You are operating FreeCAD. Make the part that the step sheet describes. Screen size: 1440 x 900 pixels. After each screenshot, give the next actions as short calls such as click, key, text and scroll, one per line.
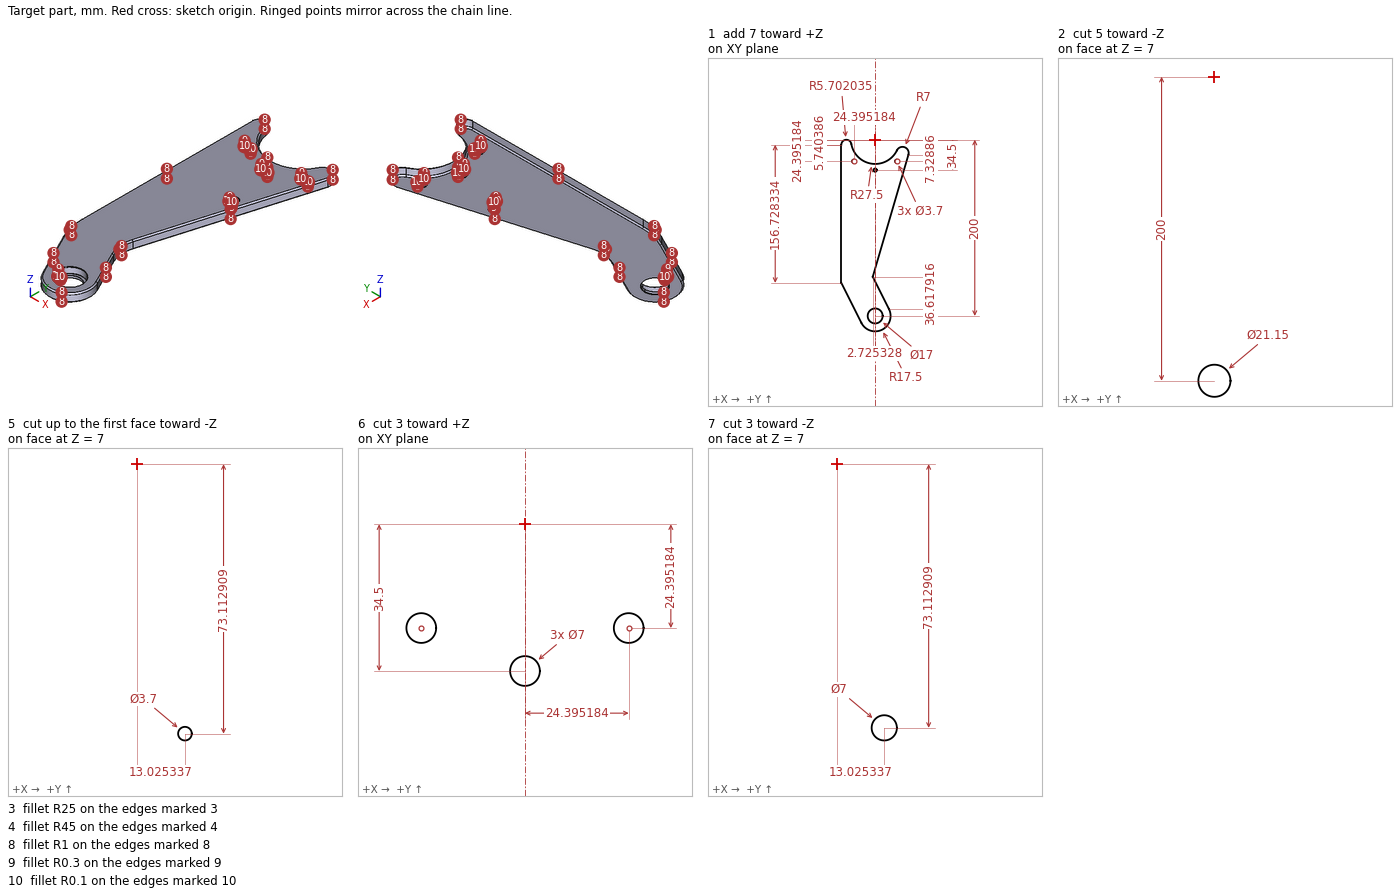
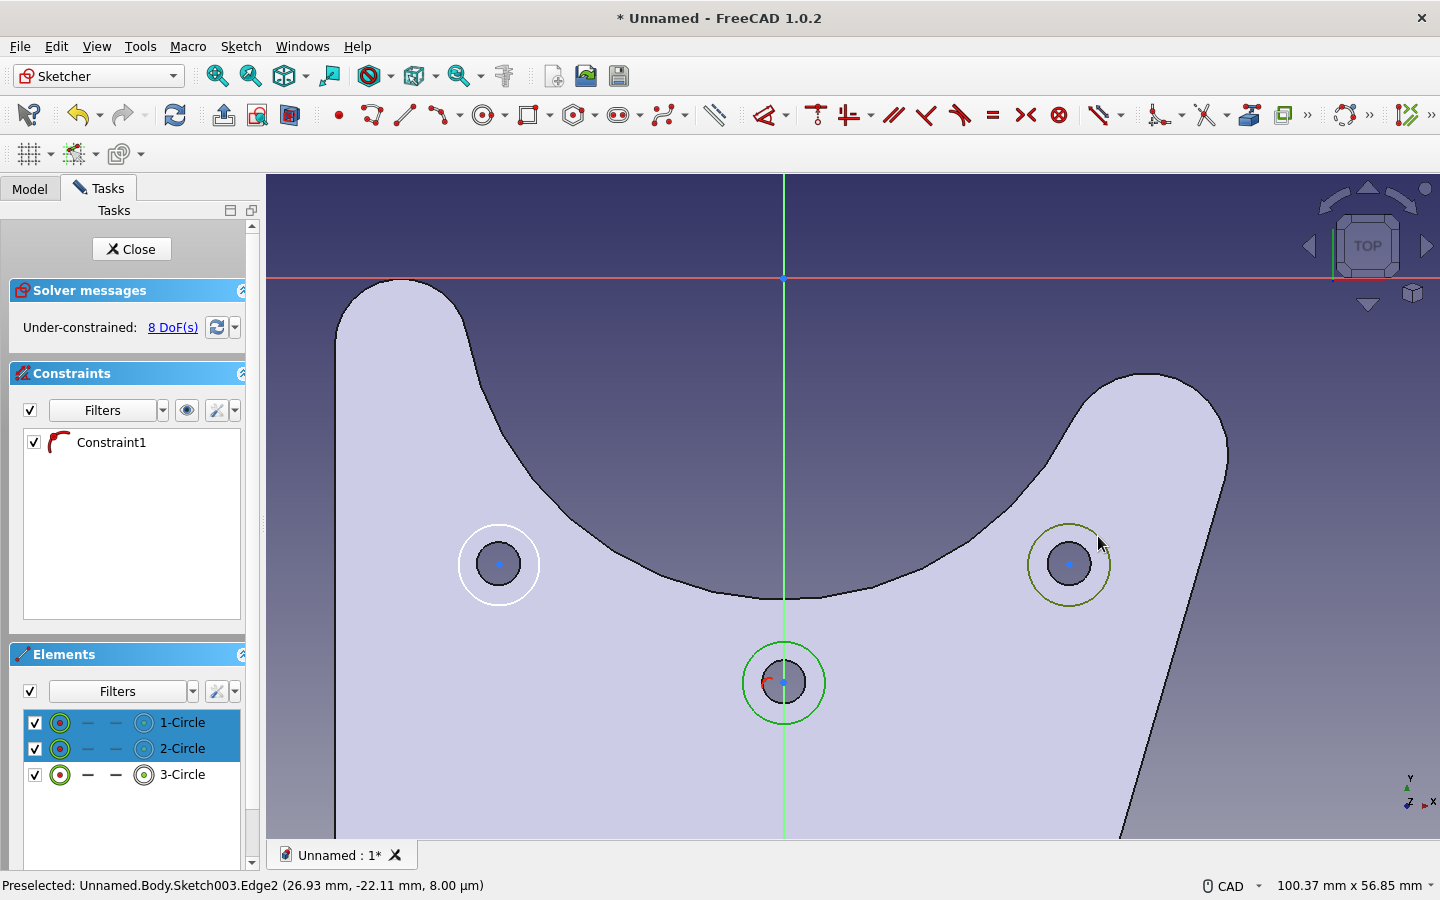
click(527, 536)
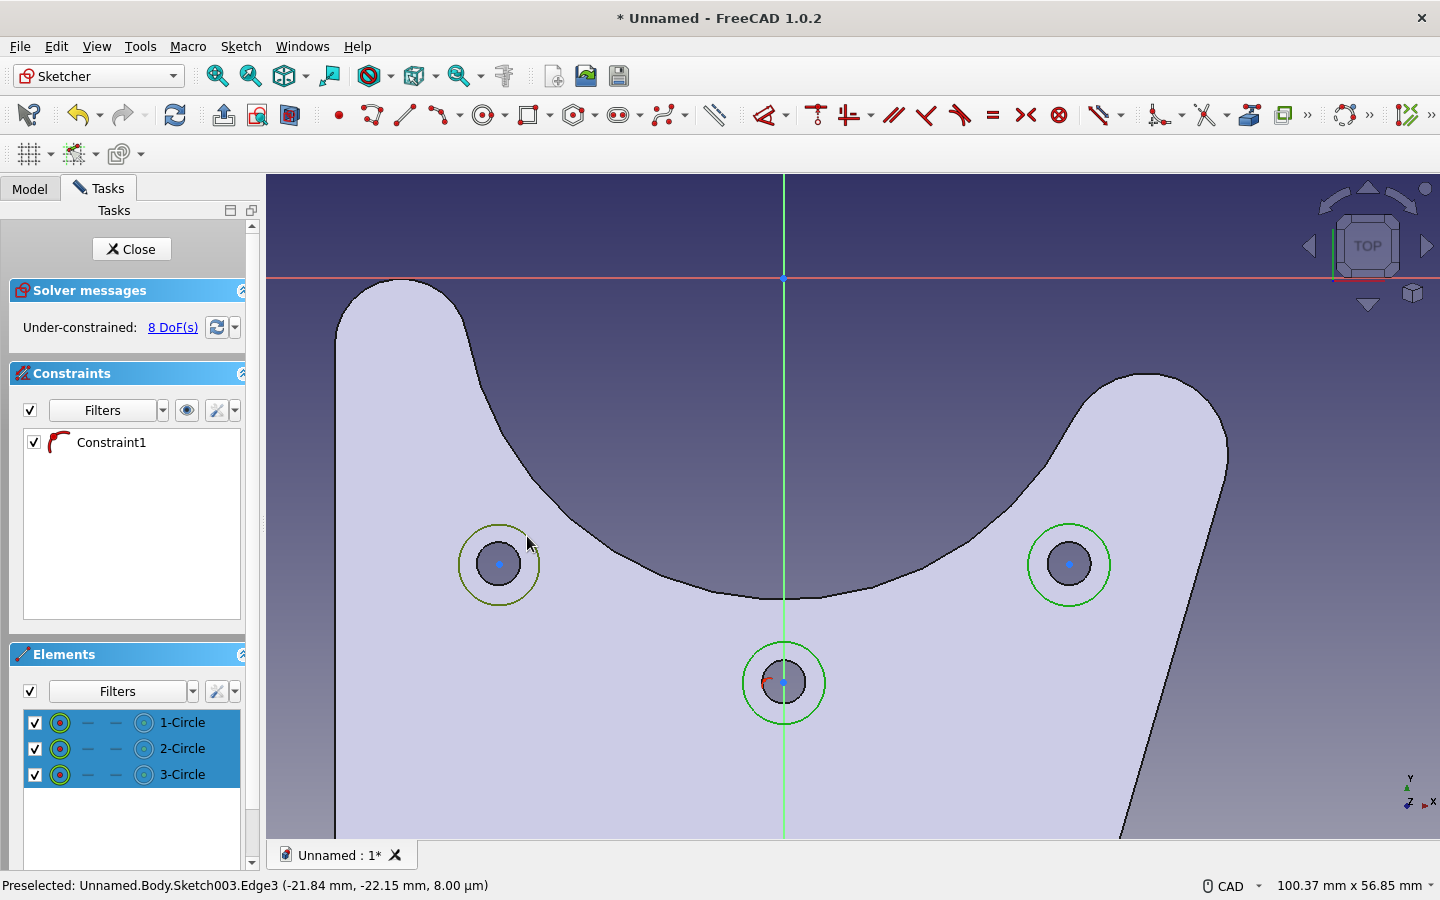
click(993, 116)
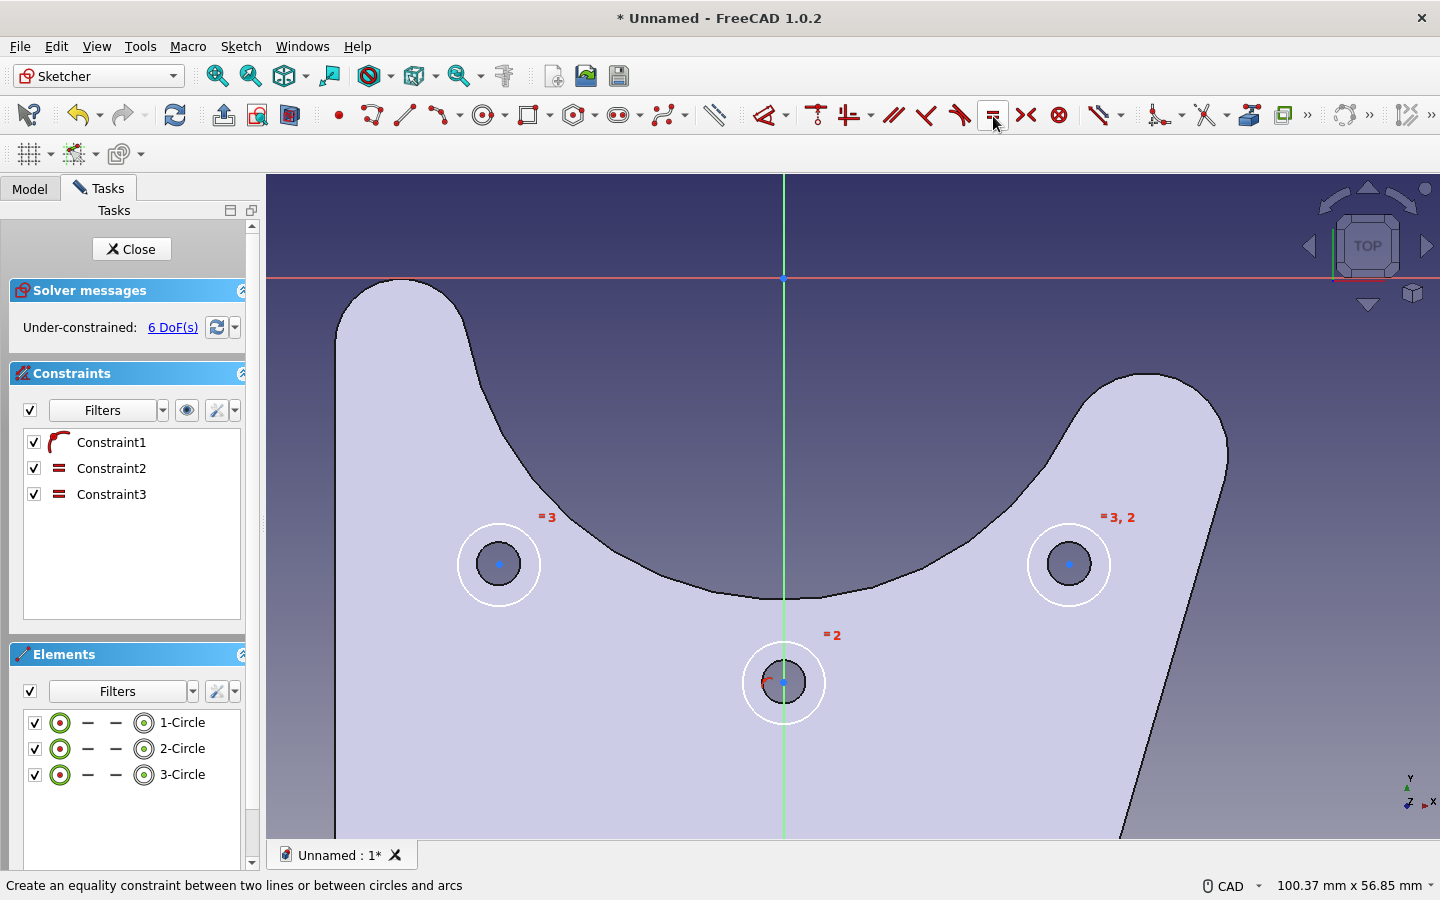
click(1069, 565)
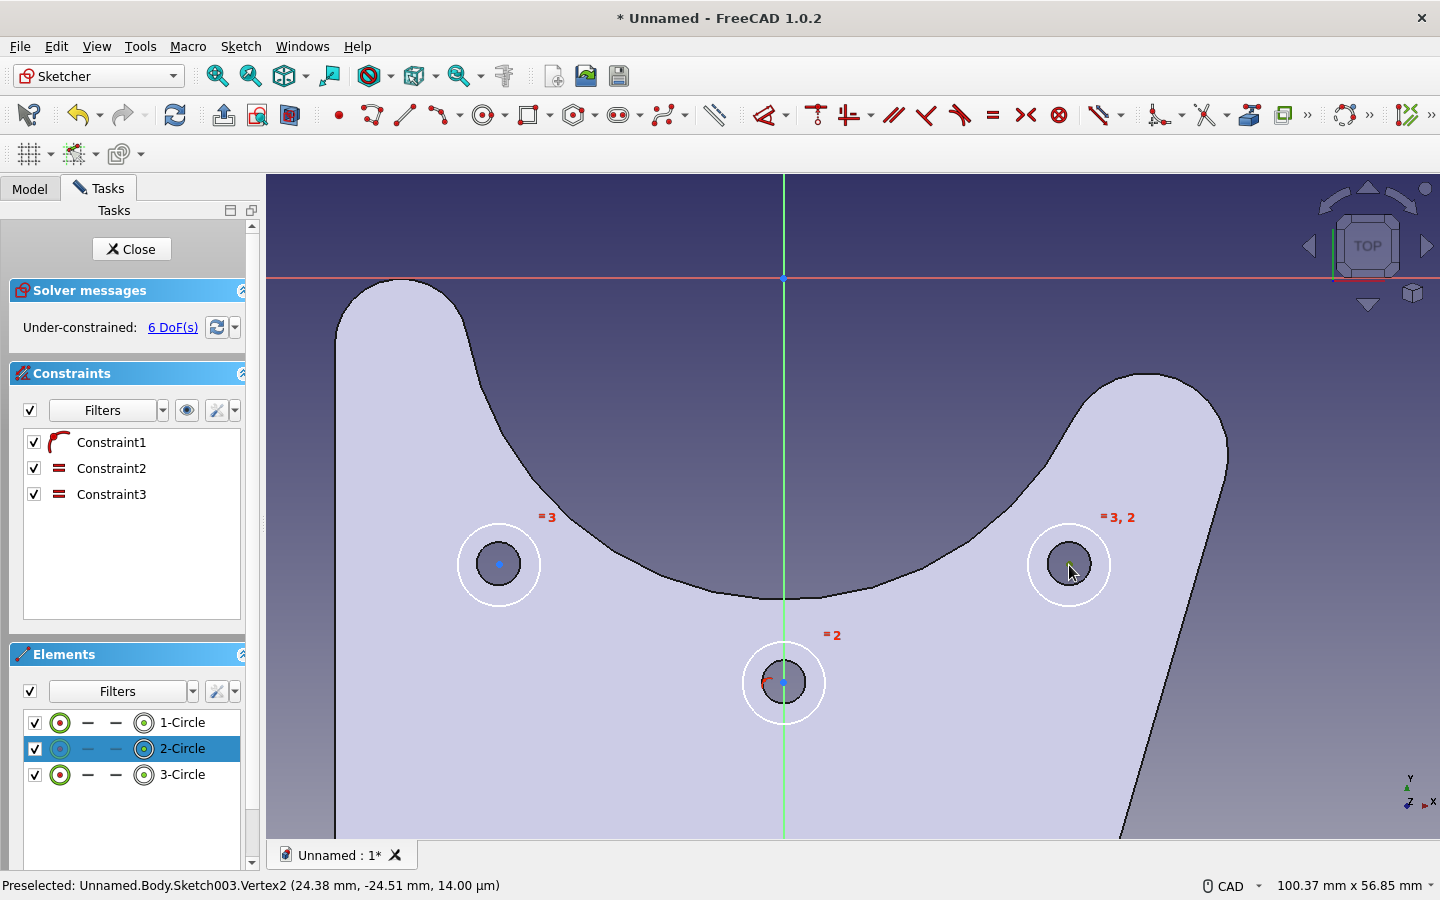
click(499, 565)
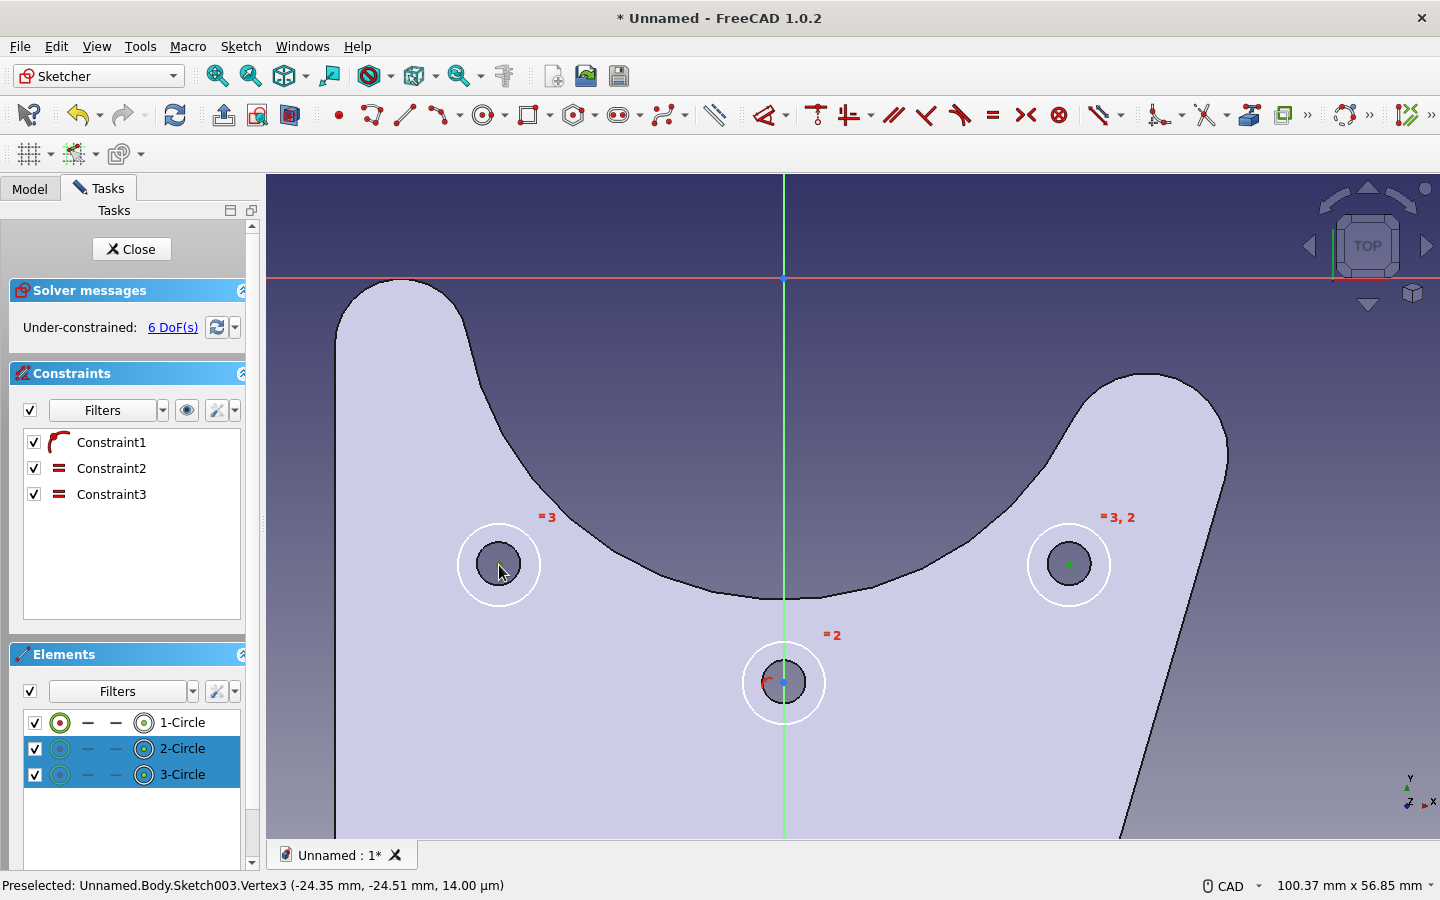
click(784, 767)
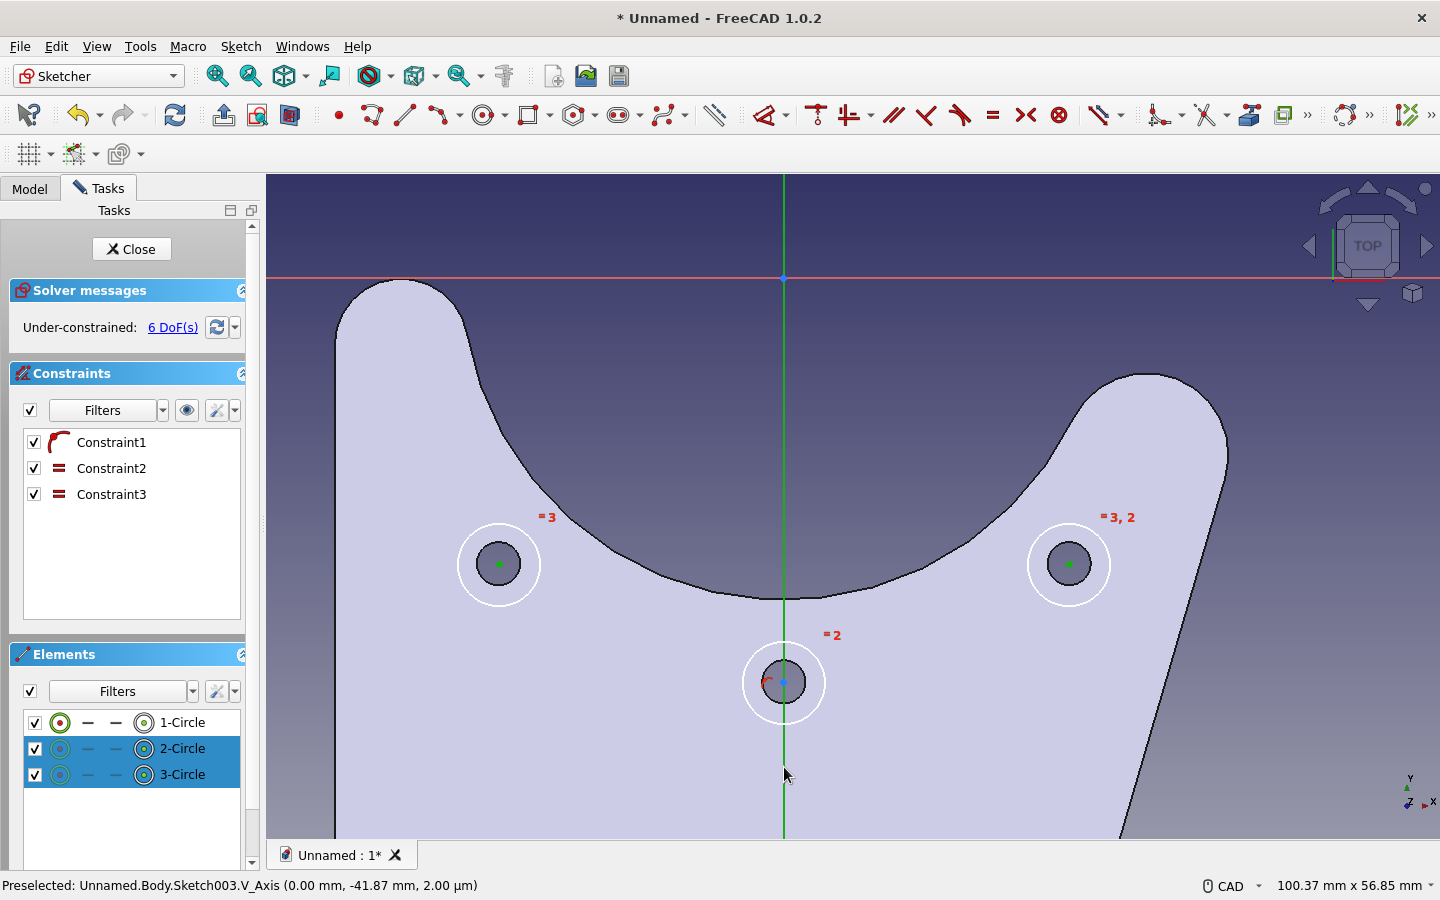
key(s)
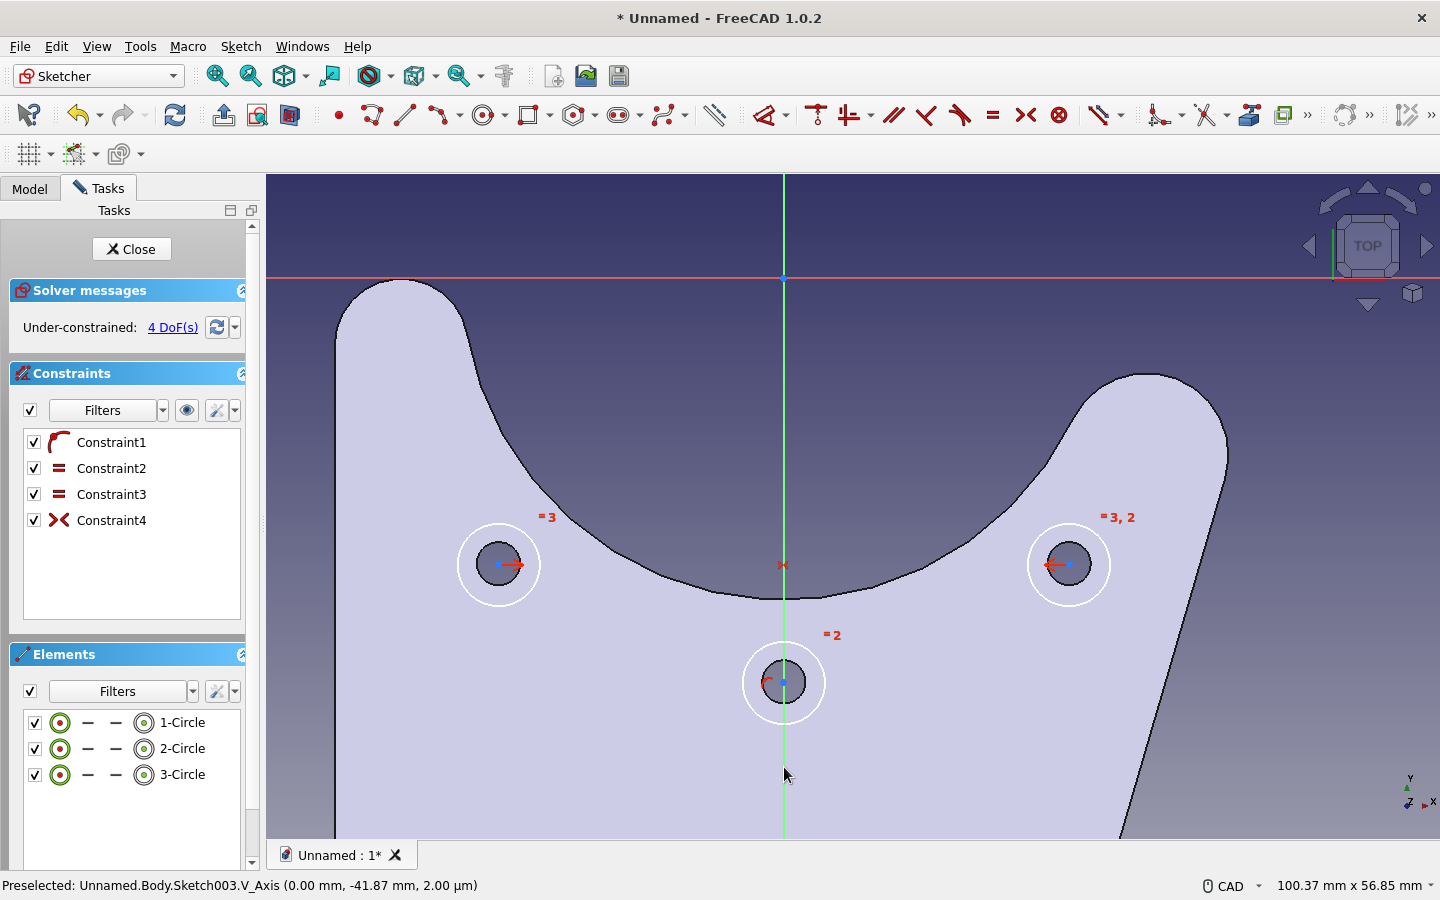
click(764, 116)